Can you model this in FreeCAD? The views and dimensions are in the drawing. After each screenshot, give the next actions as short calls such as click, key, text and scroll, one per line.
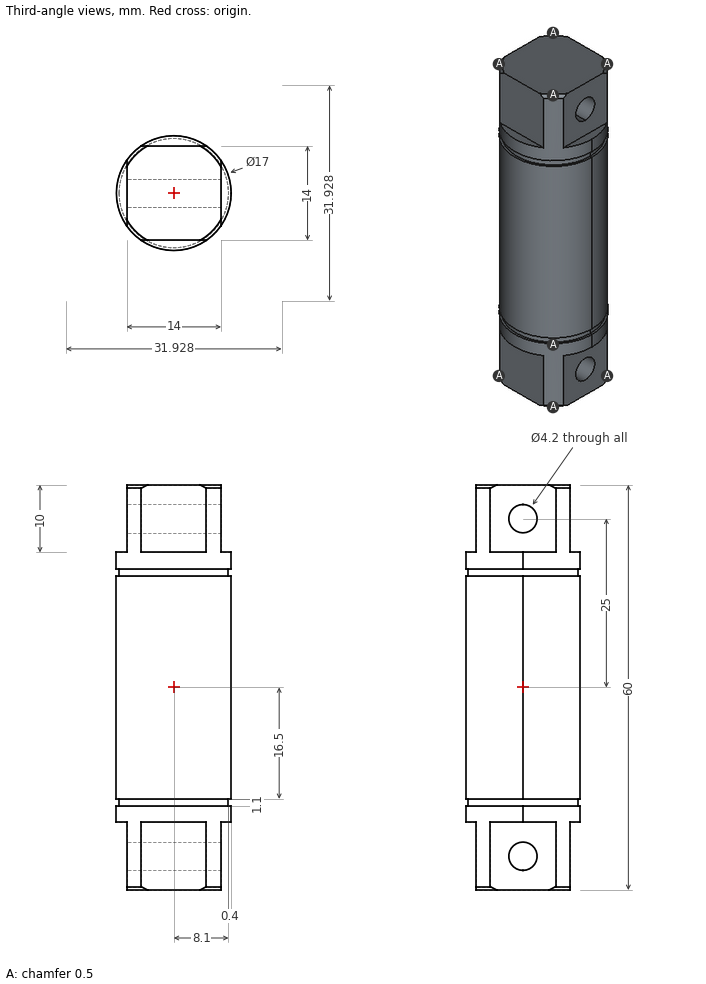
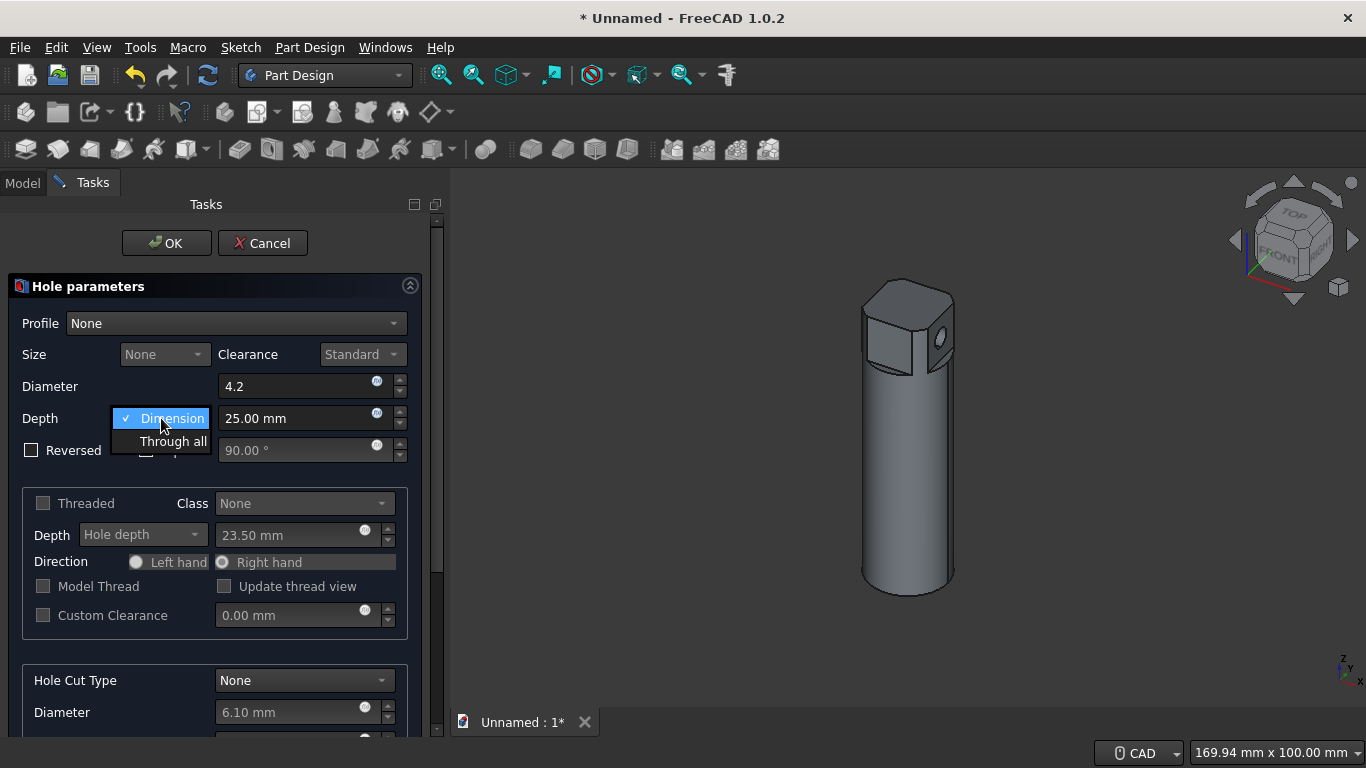
click(160, 442)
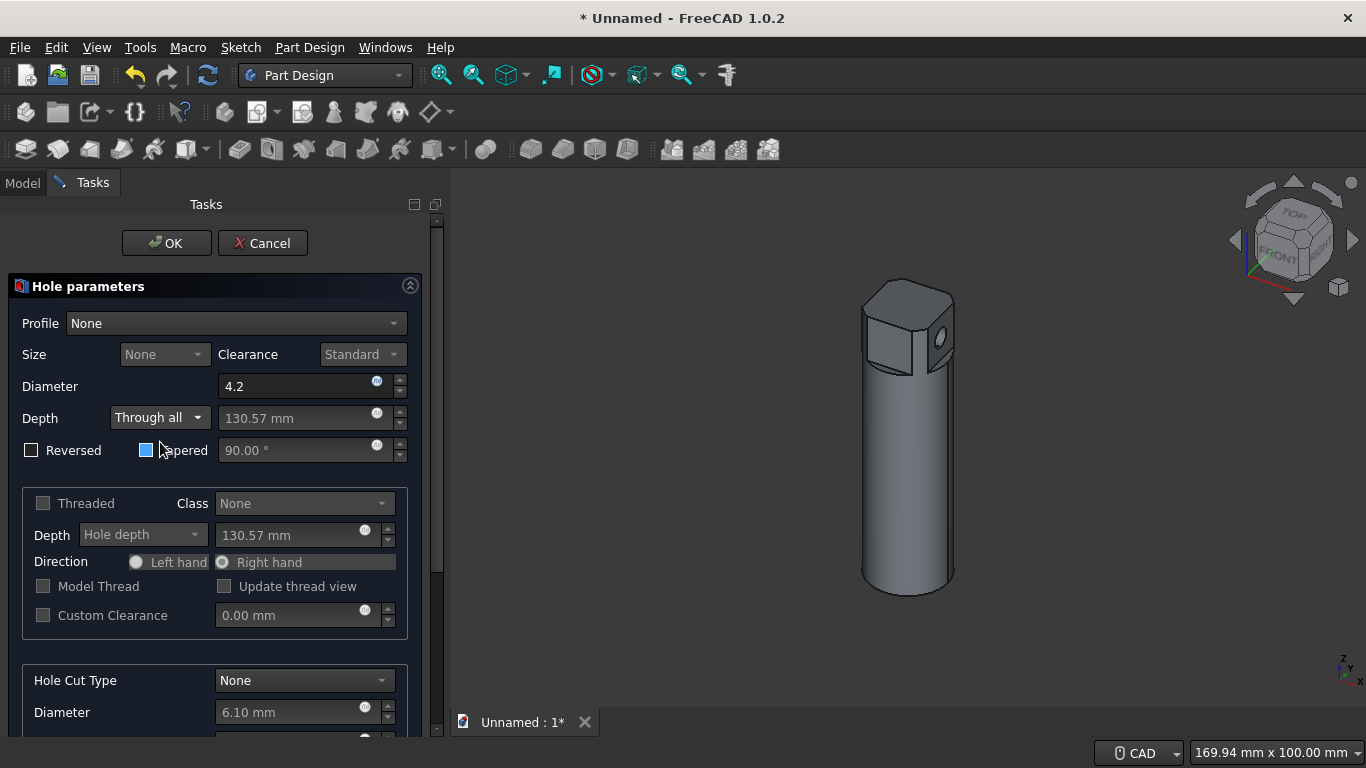
click(167, 243)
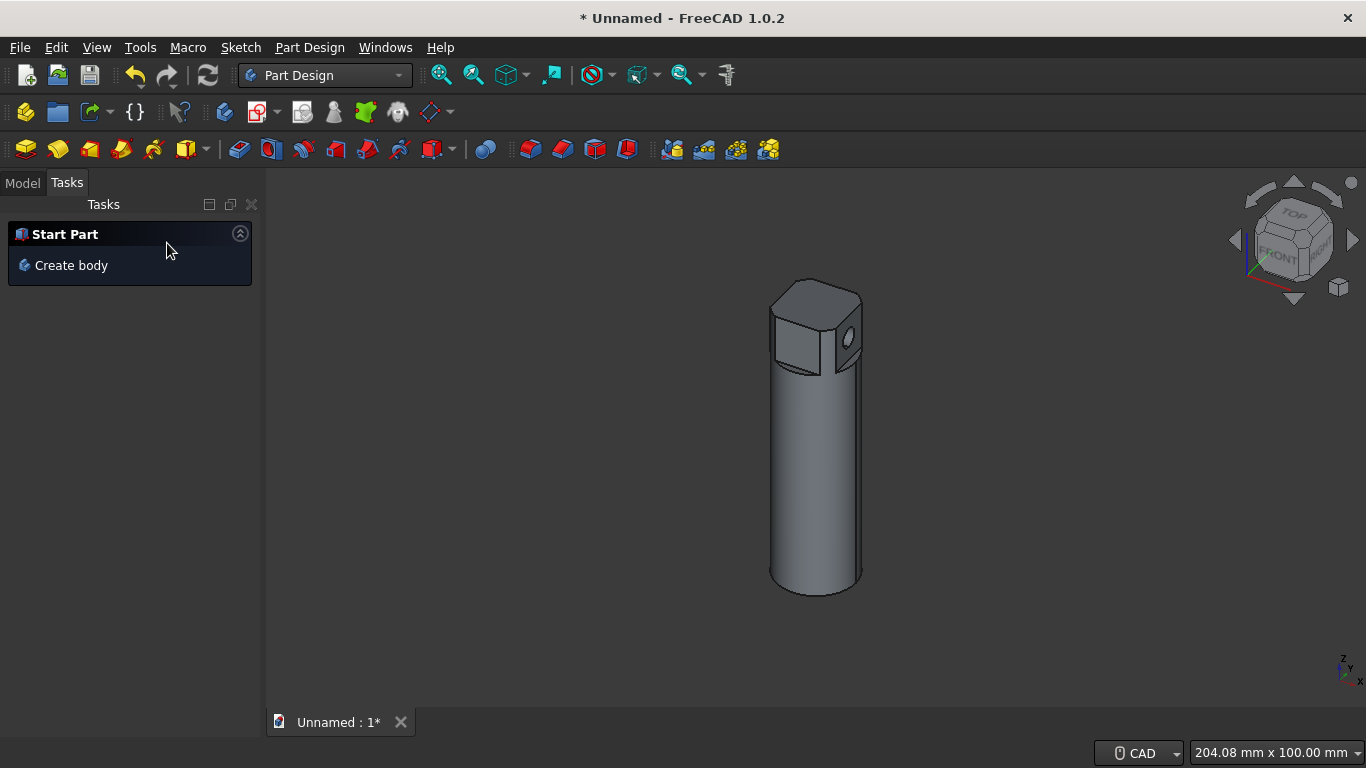
click(23, 182)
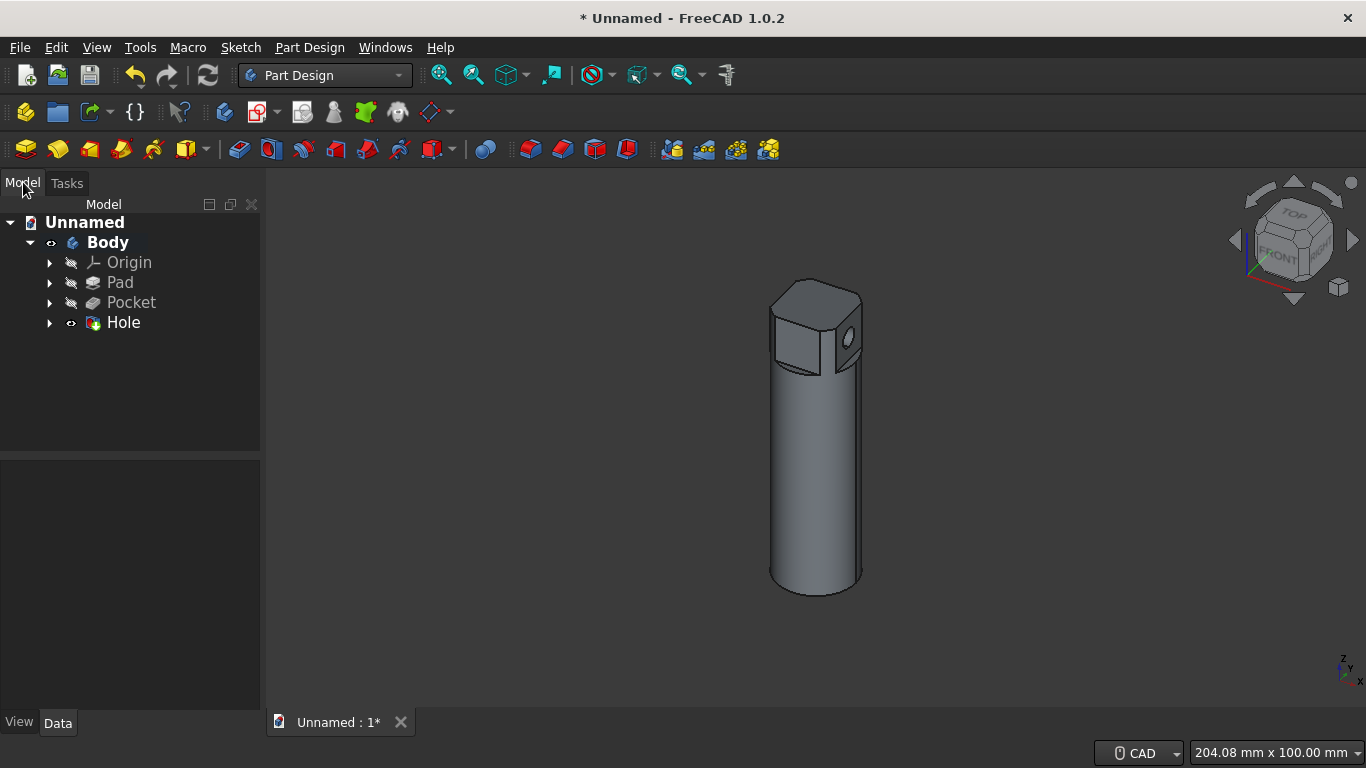
click(116, 303)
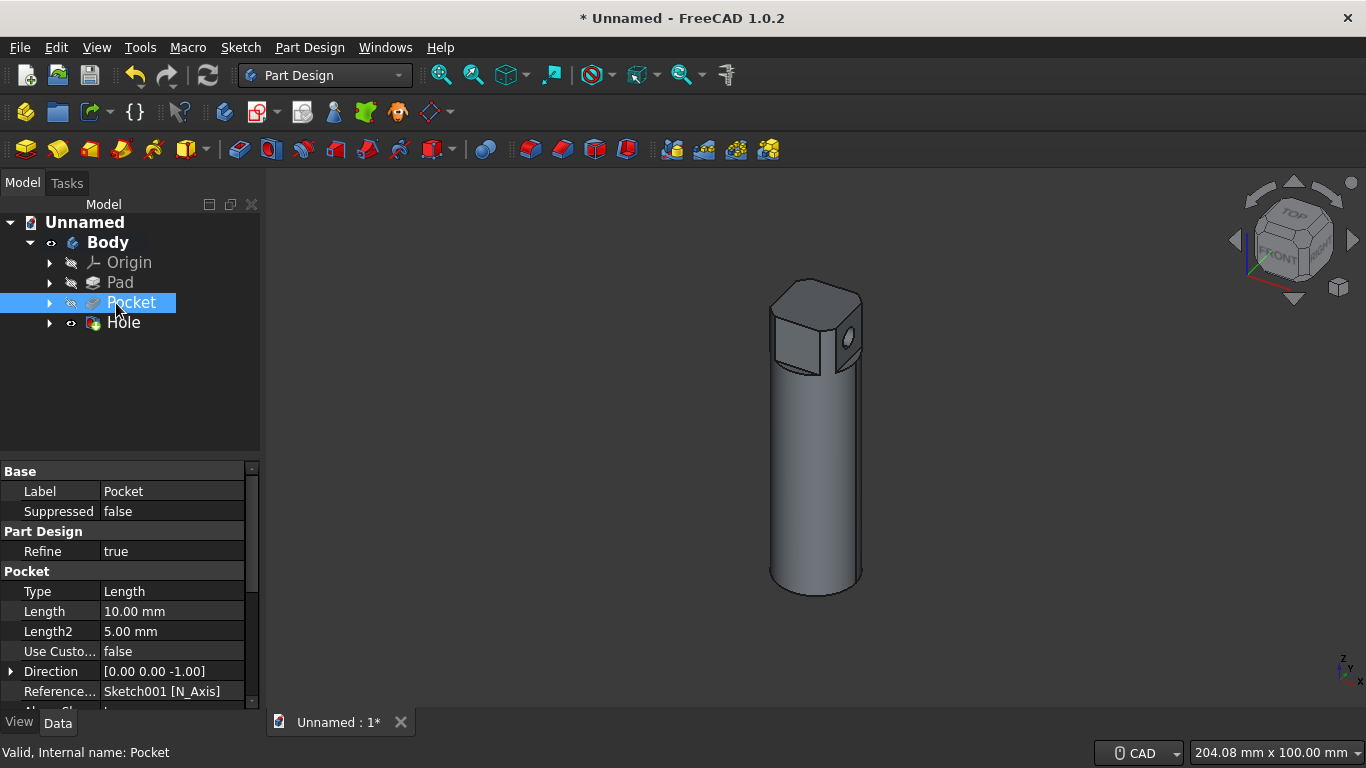
click(116, 323, ctrl)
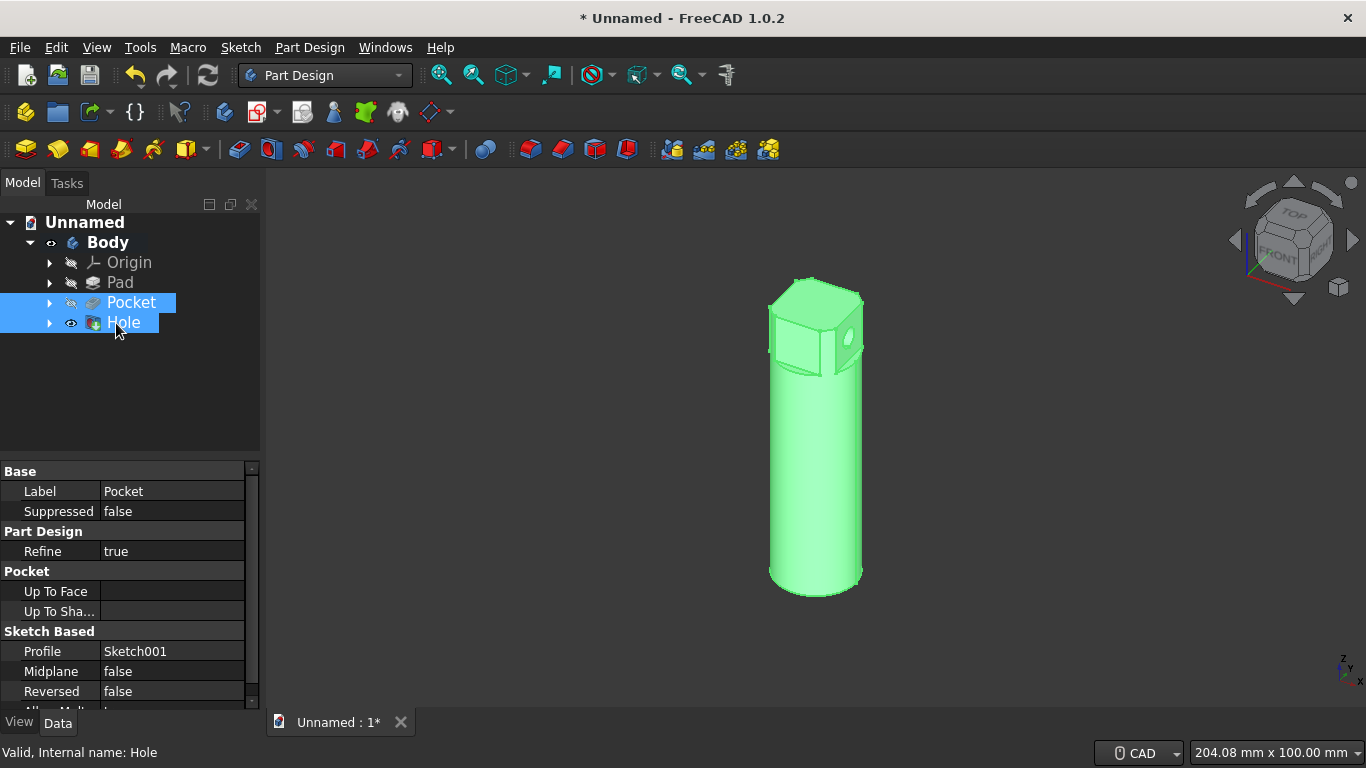
click(672, 150)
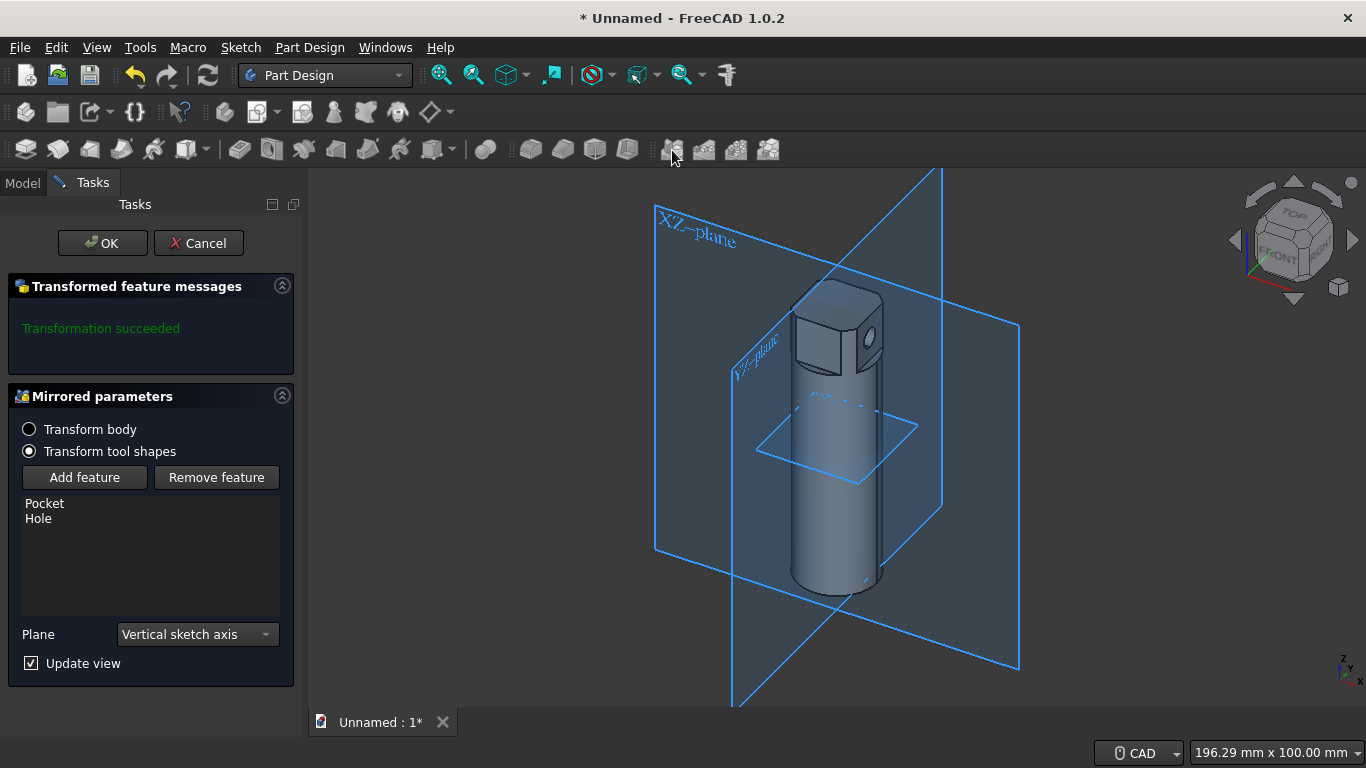
click(198, 634)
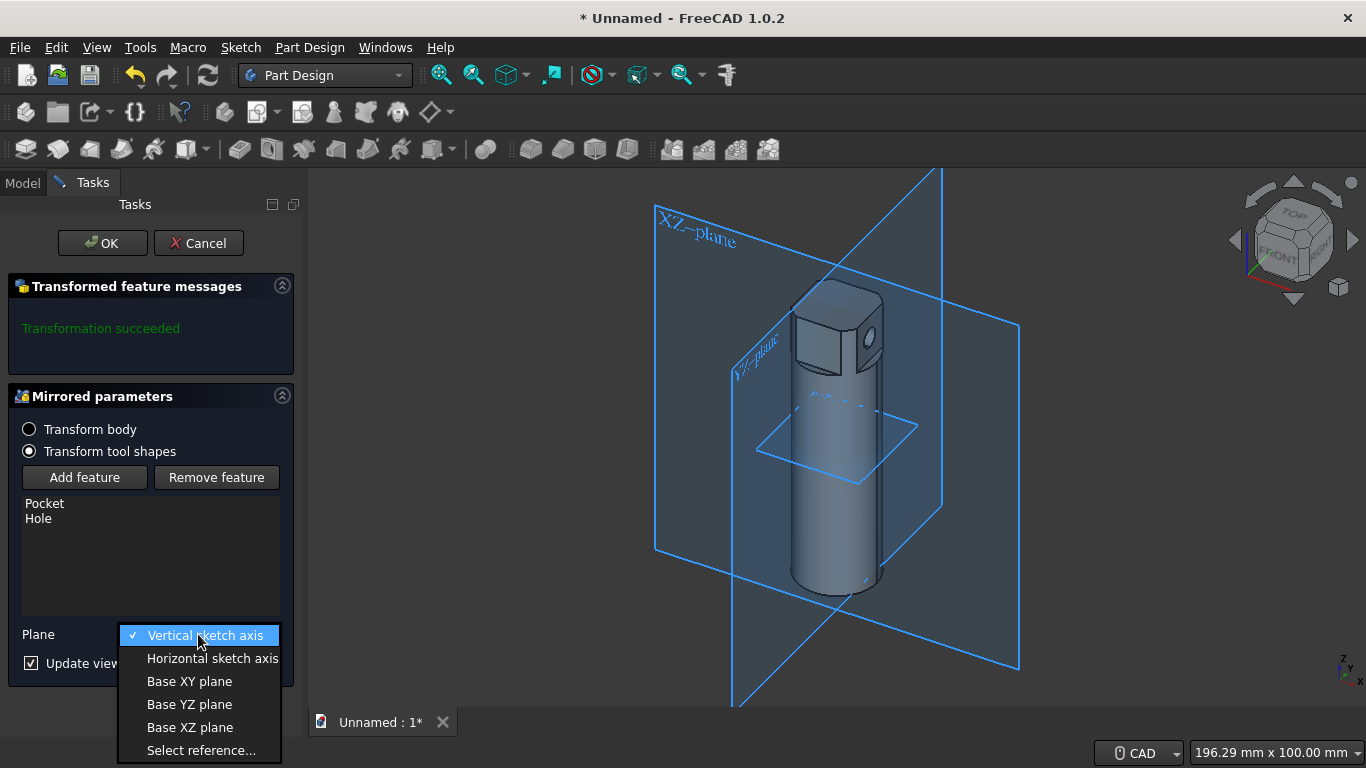
click(198, 682)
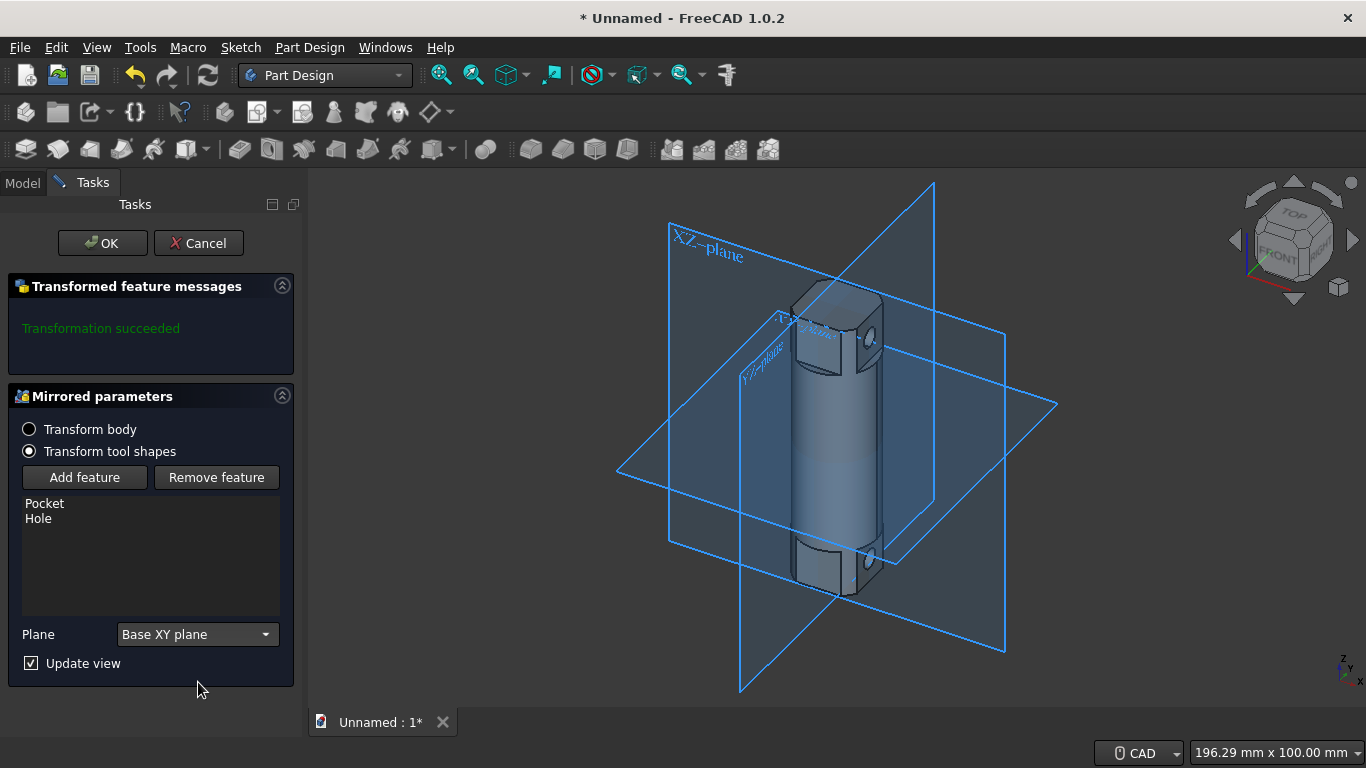
click(103, 243)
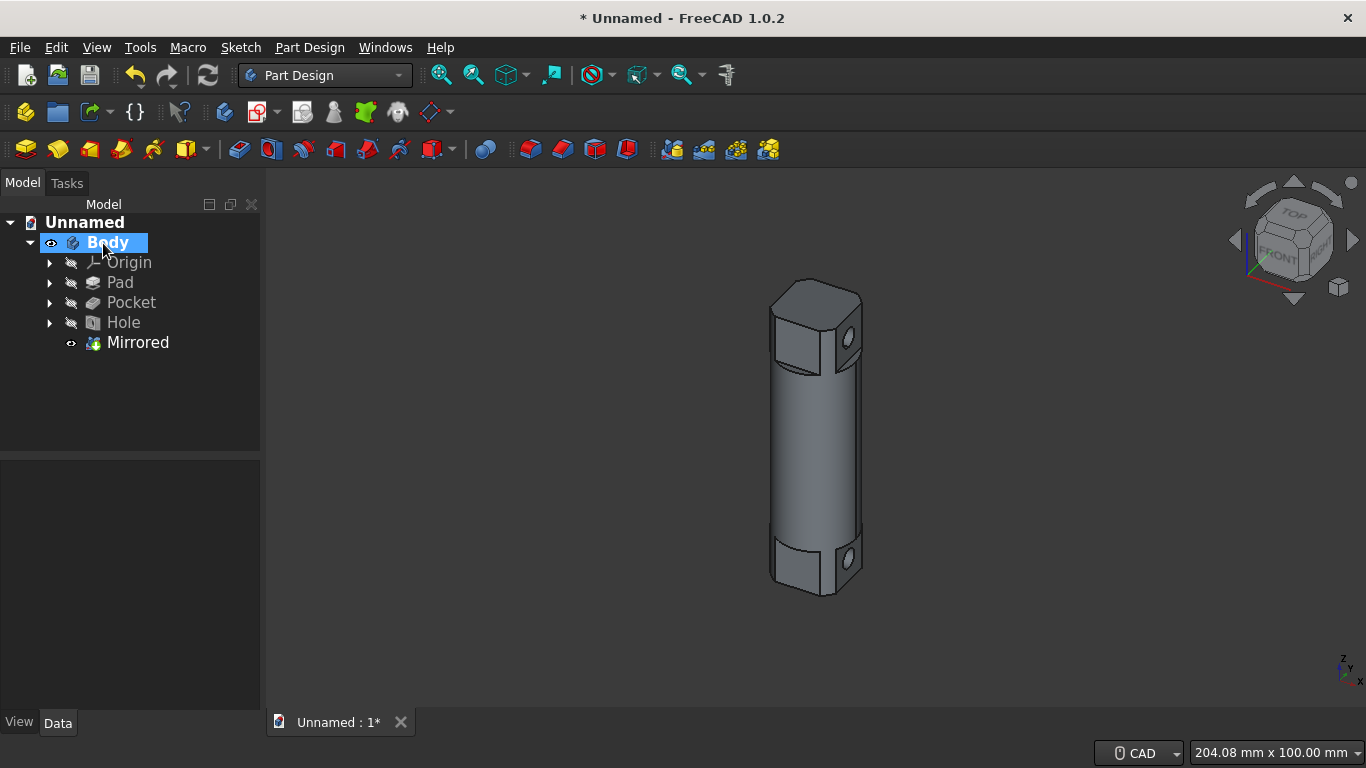
click(771, 310)